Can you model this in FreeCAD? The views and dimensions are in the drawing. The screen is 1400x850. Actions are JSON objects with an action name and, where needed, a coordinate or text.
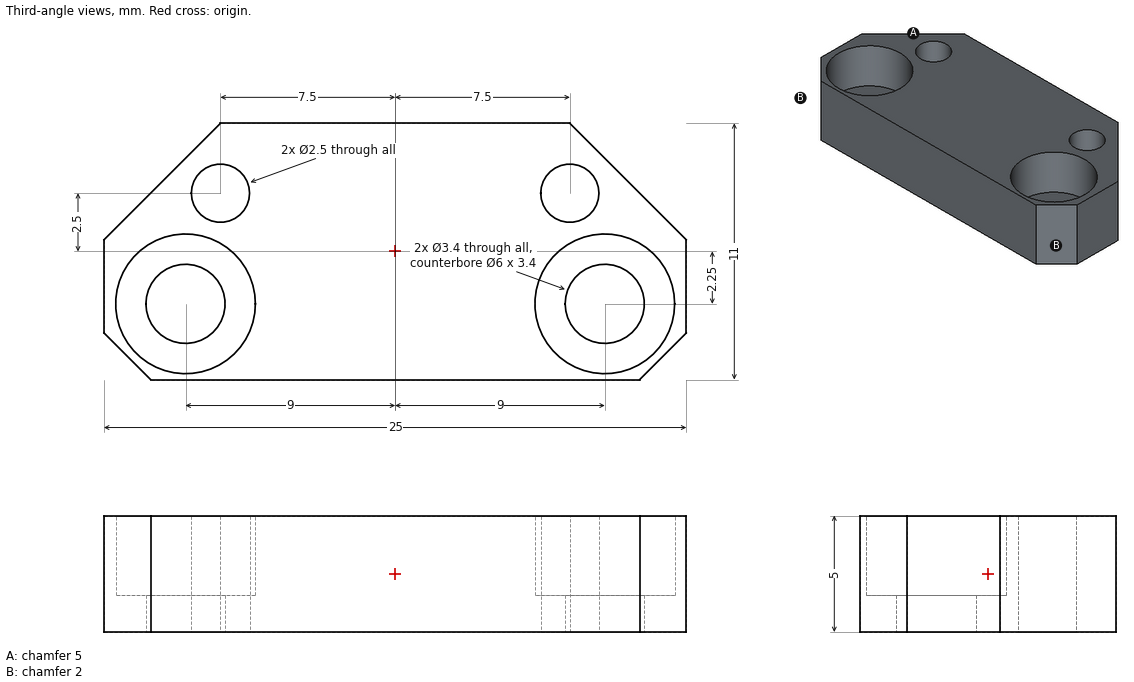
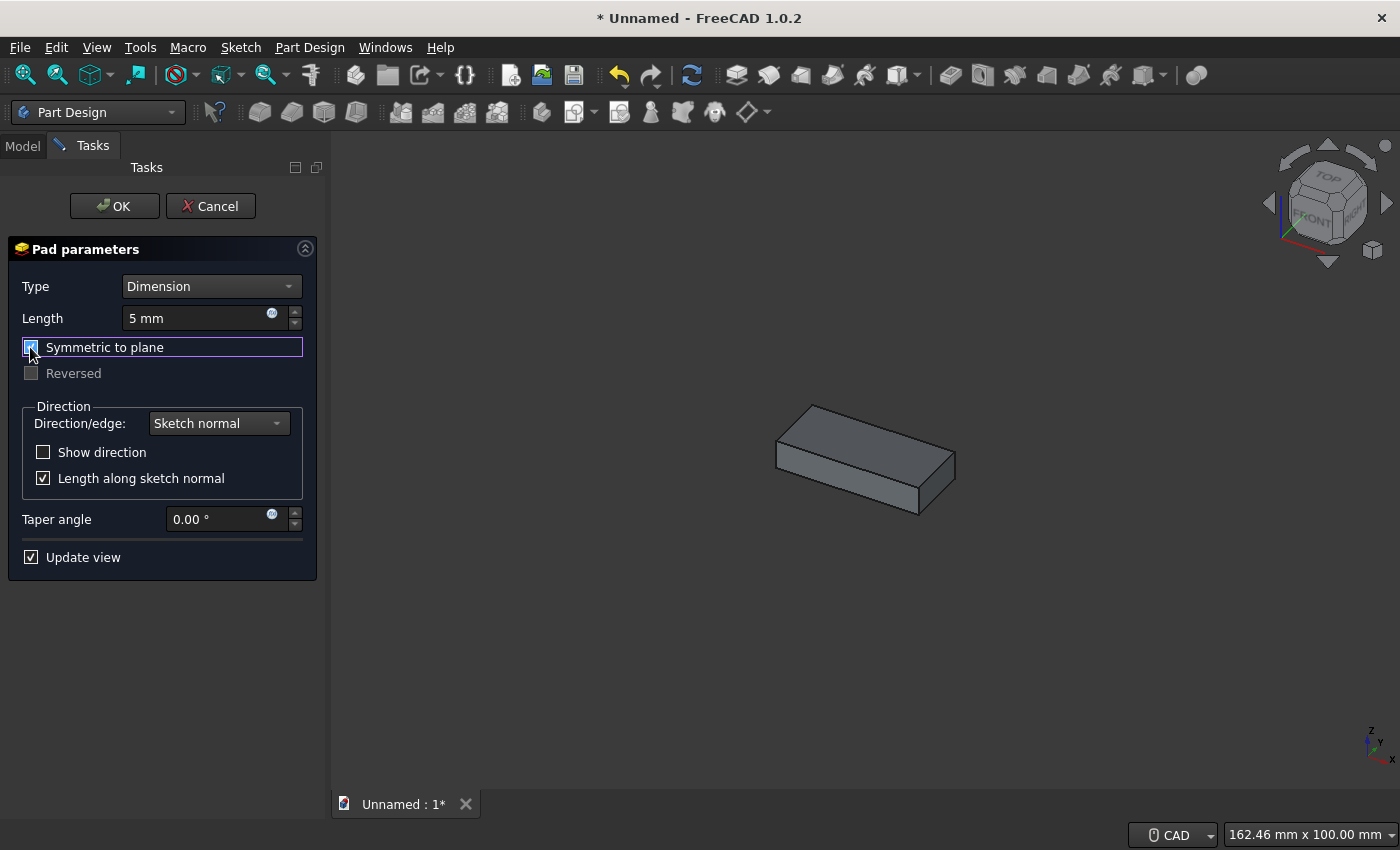
{"action": "left_click", "coordinate": [115, 206]}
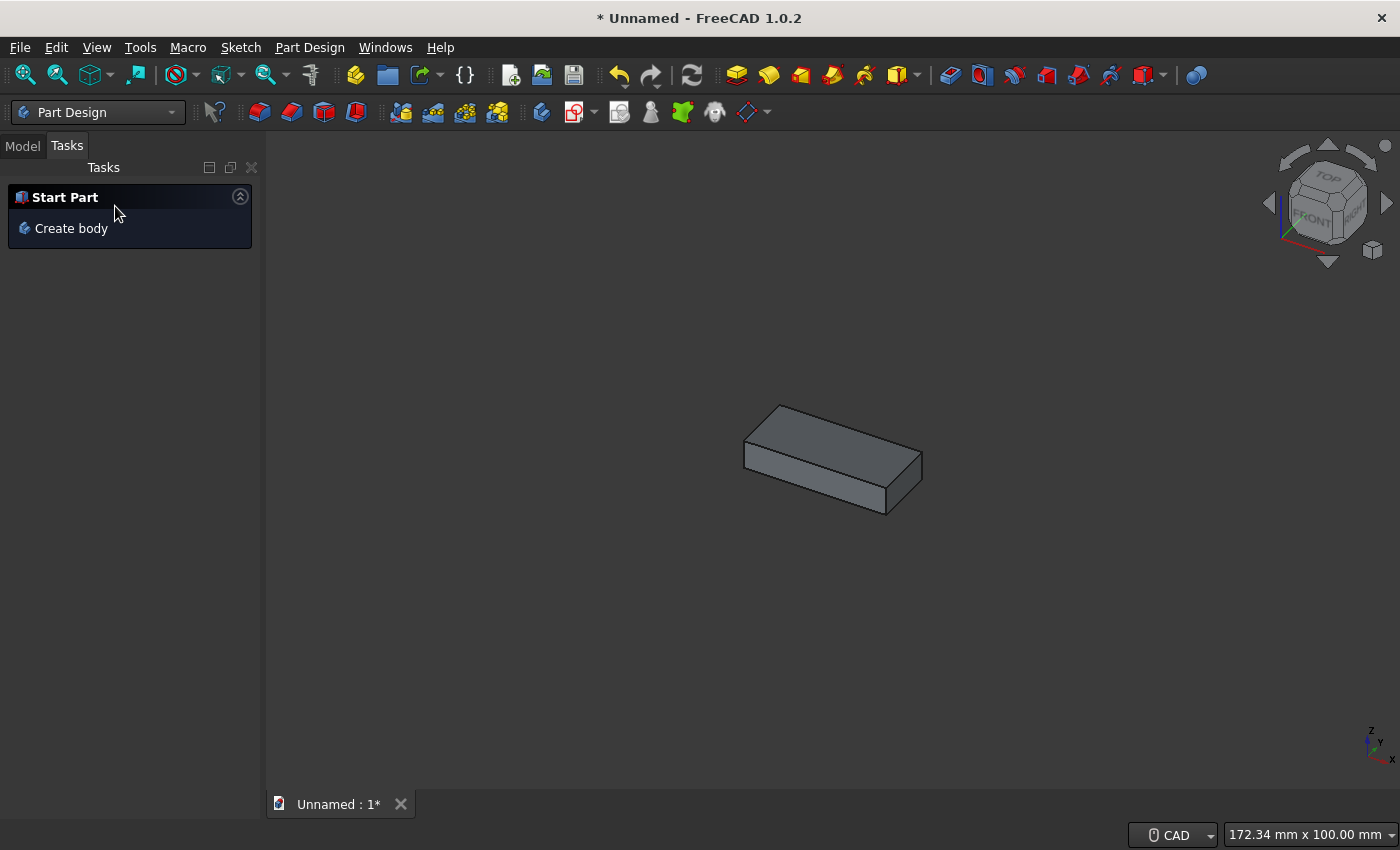
{"action": "left_click", "coordinate": [26, 76]}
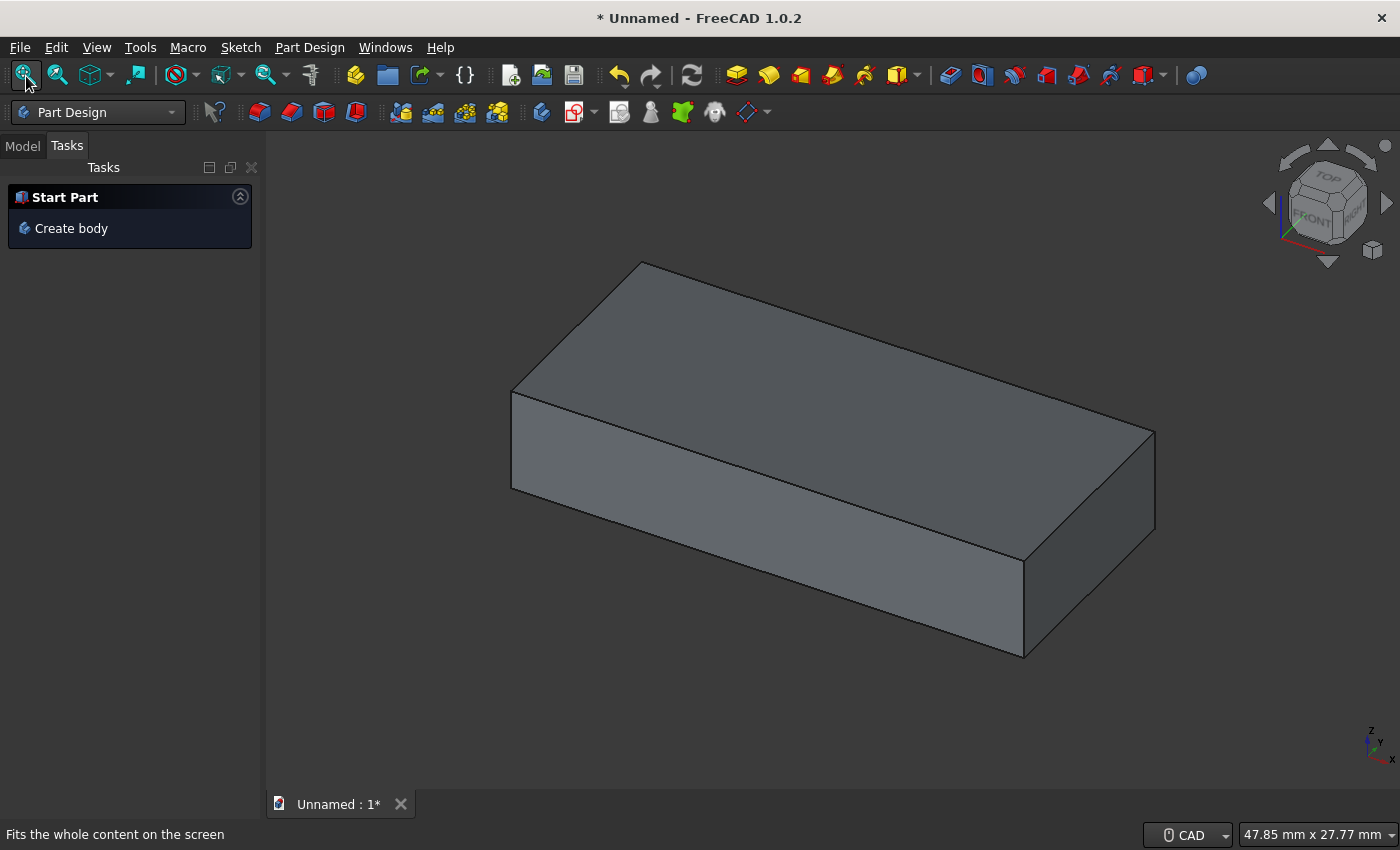
{"action": "left_click", "coordinate": [906, 435]}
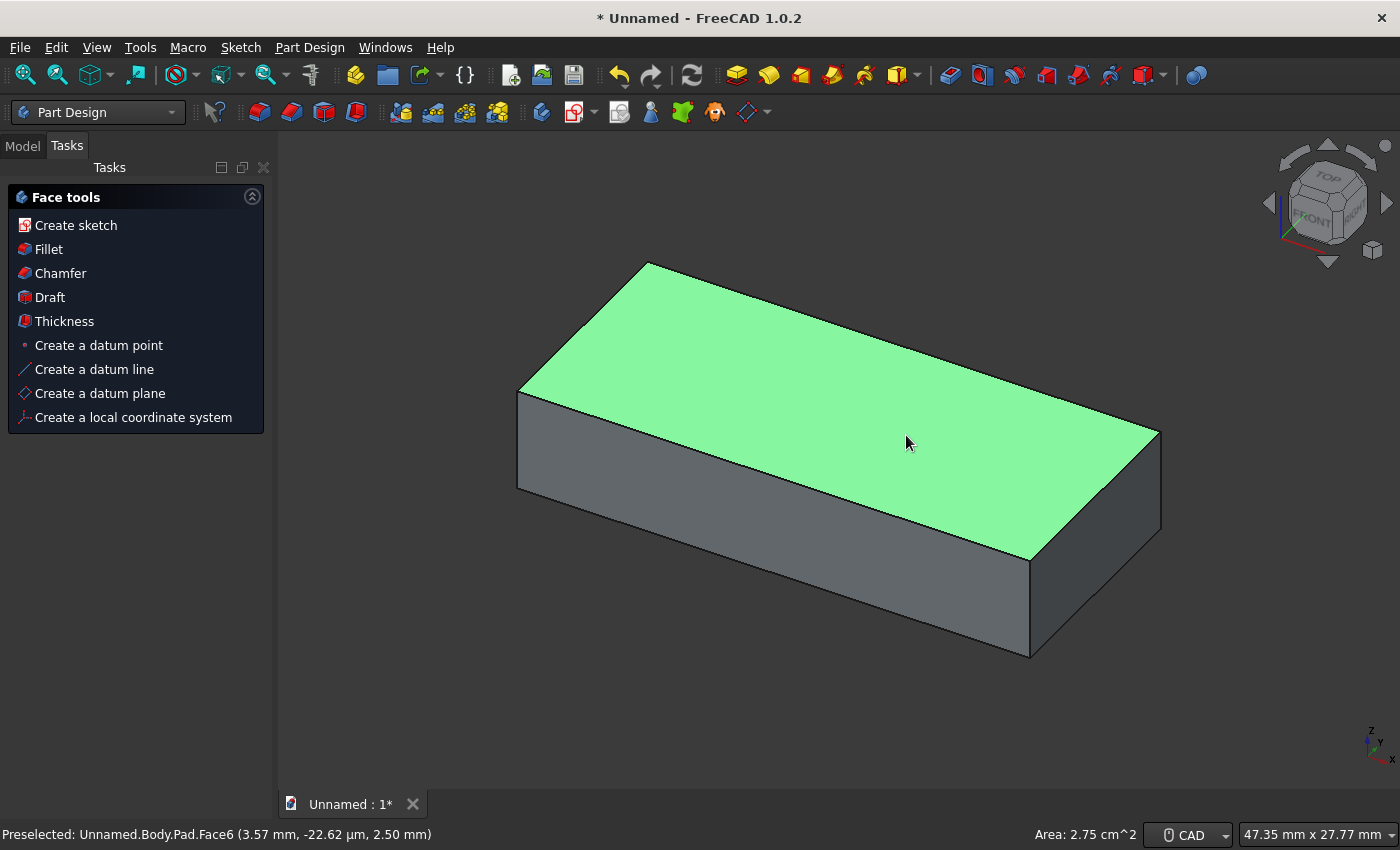
{"action": "left_click", "coordinate": [574, 112]}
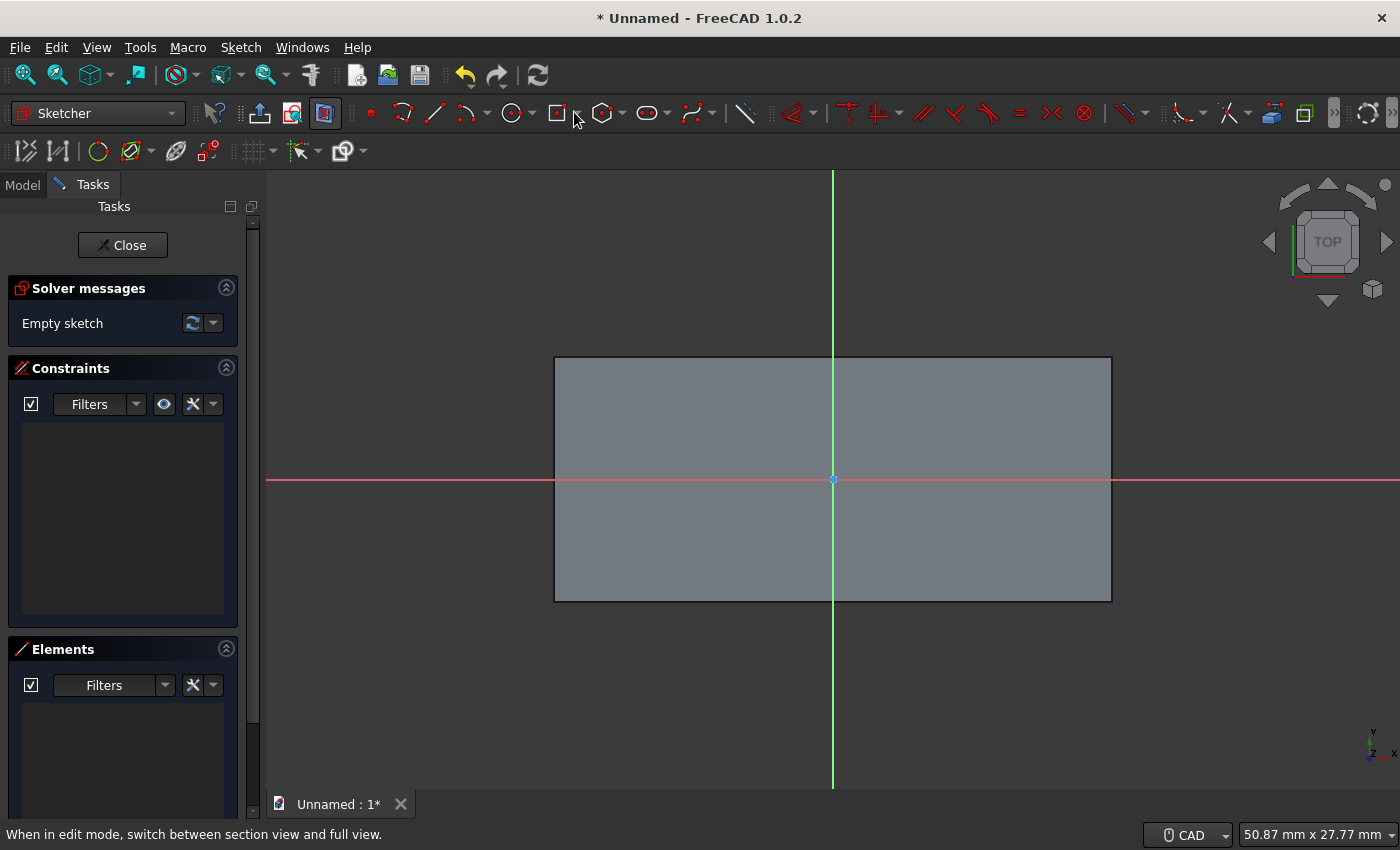
{"action": "scroll", "coordinate": [916, 387], "scroll_direction": "up", "scroll_amount": 3}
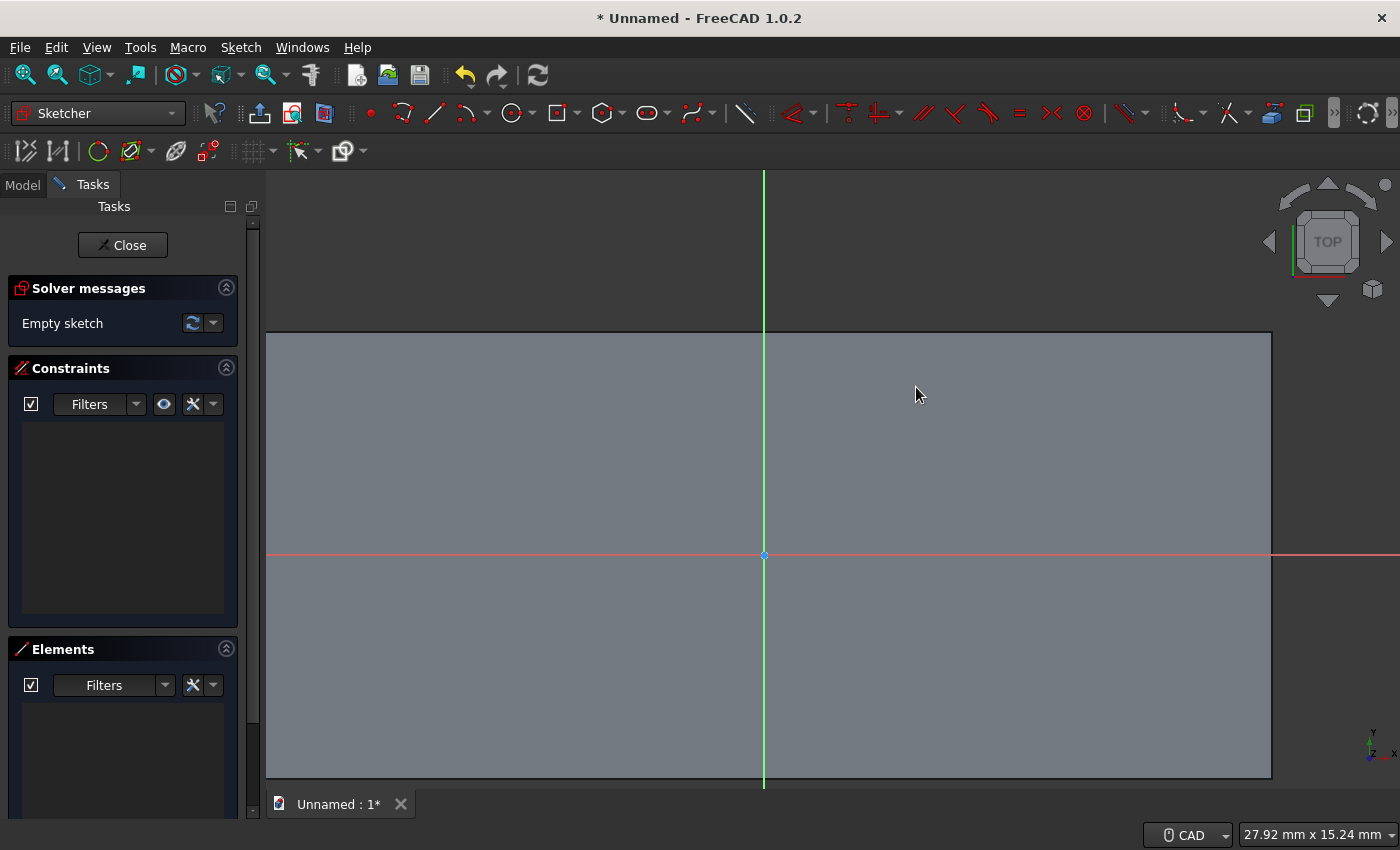
{"action": "key", "text": "g c"}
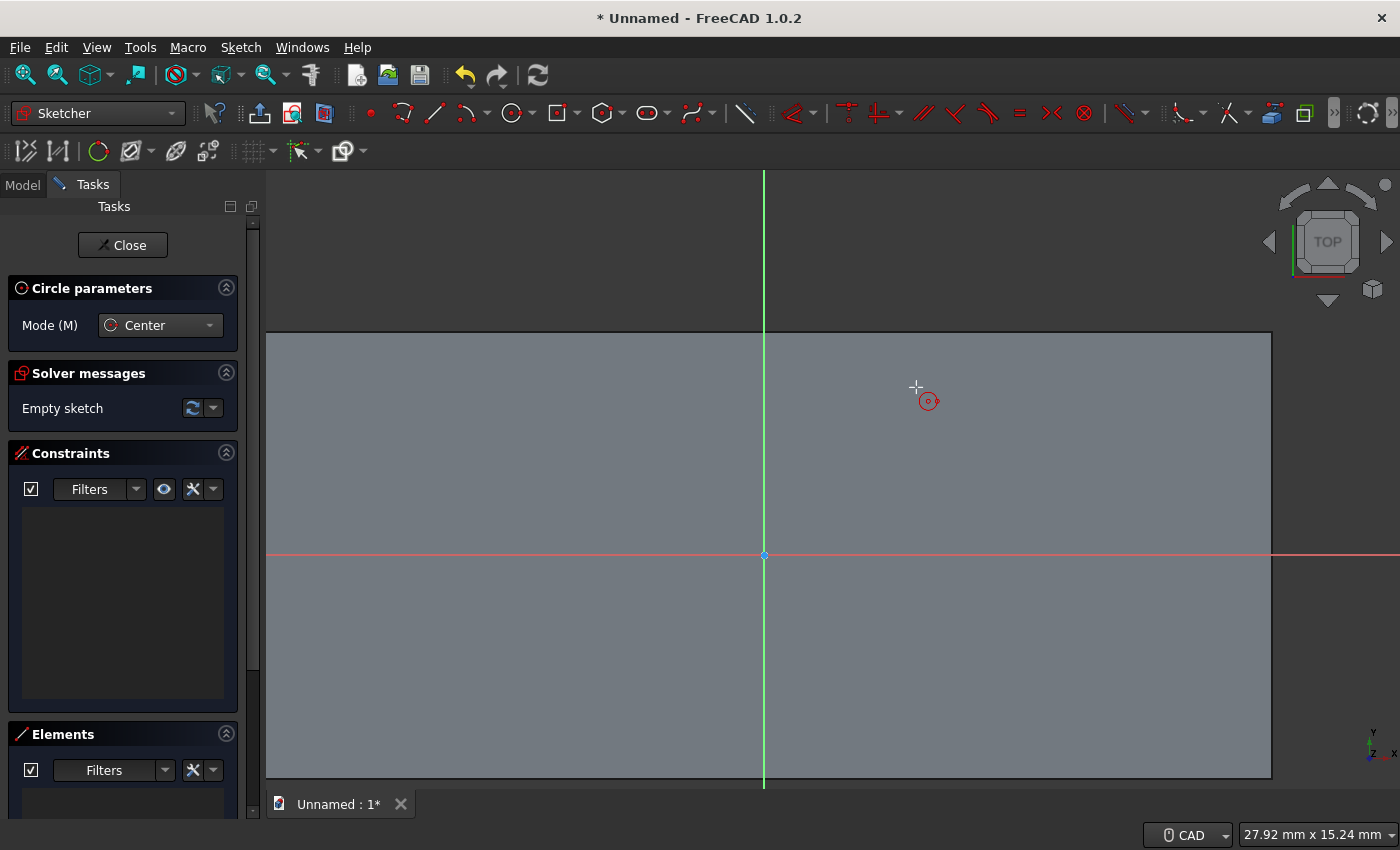
{"action": "left_click", "coordinate": [460, 454]}
{"action": "left_click", "coordinate": [496, 418]}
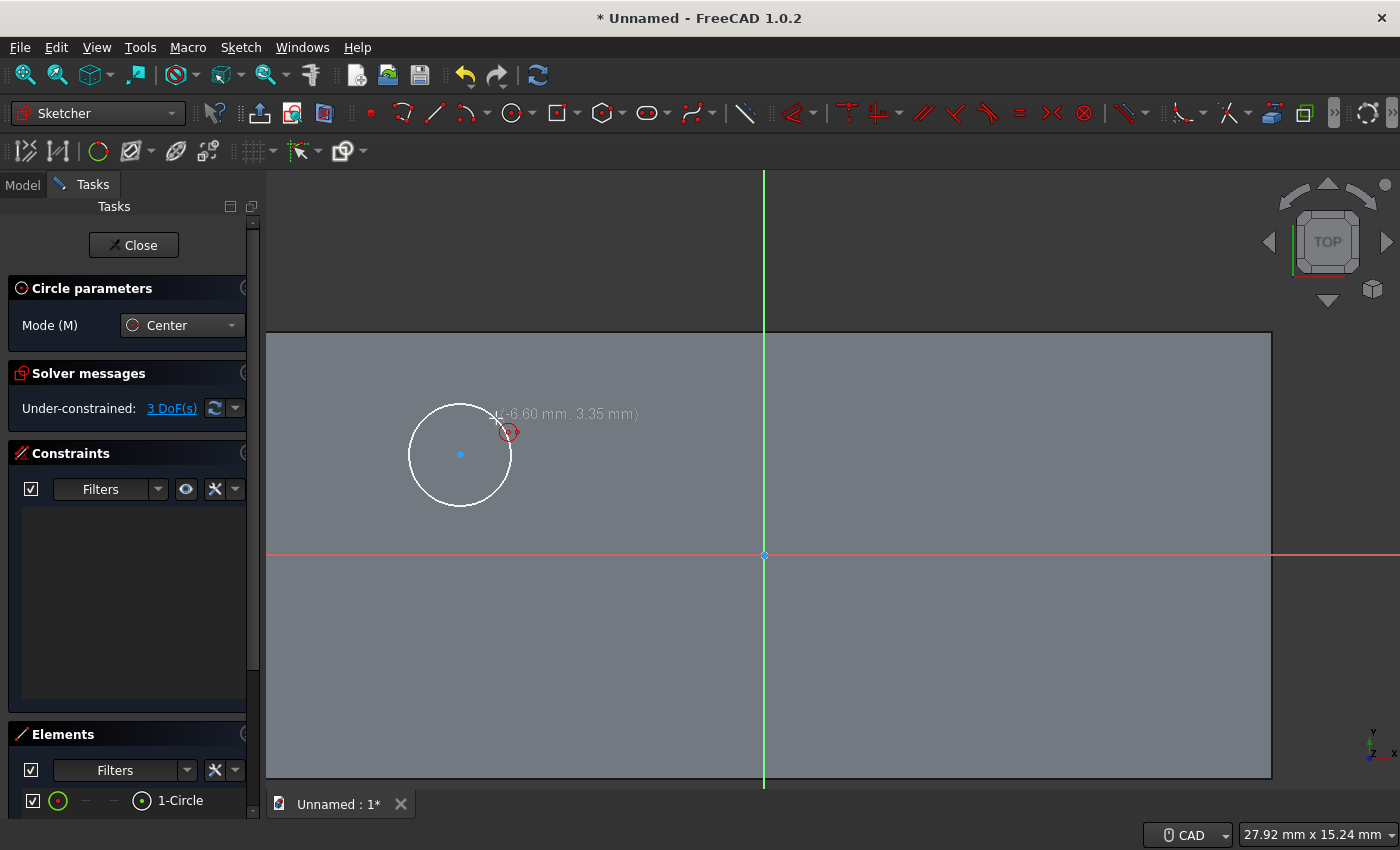
{"action": "left_click", "coordinate": [1069, 454]}
{"action": "left_click", "coordinate": [1105, 418]}
{"action": "key", "text": "Escape"}